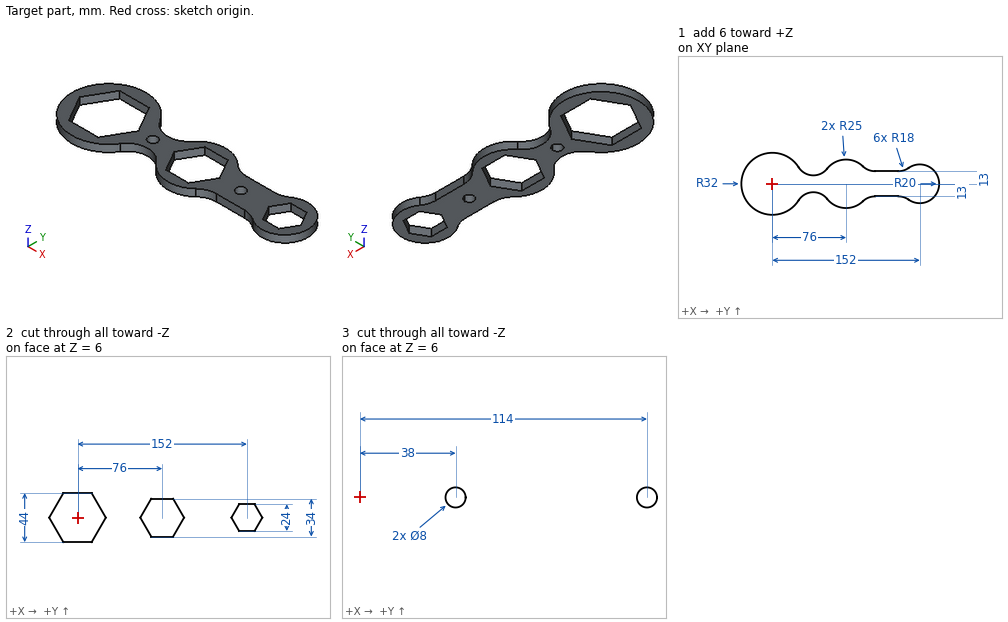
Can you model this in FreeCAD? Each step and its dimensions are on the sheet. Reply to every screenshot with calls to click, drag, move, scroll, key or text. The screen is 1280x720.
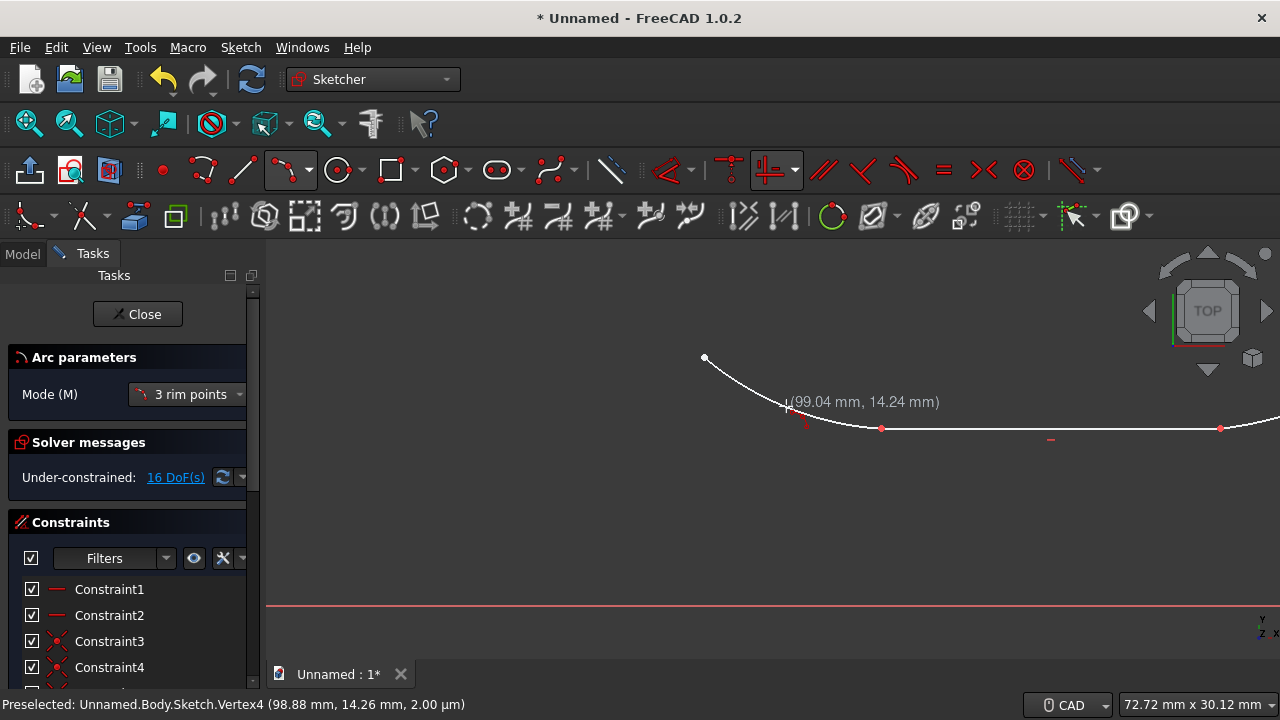
scroll(786, 409, down, 8)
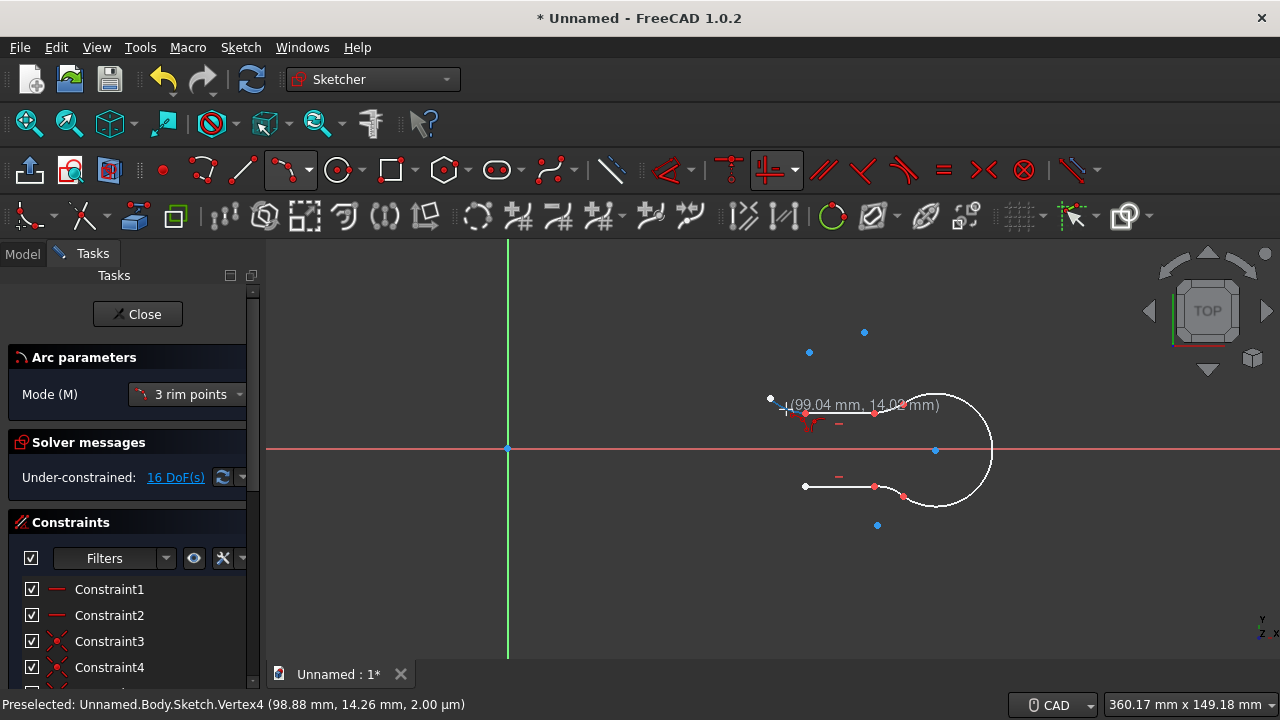
click(770, 399)
click(666, 405)
click(717, 379)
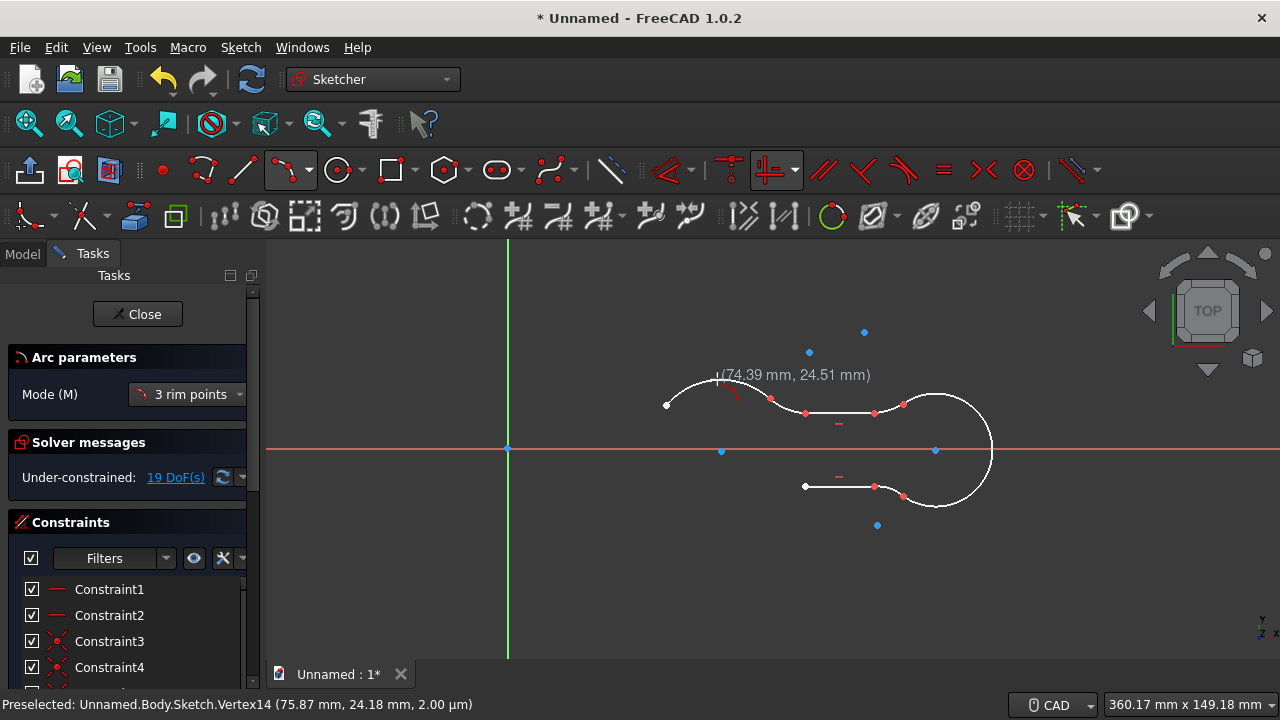
click(666, 406)
click(584, 401)
click(624, 424)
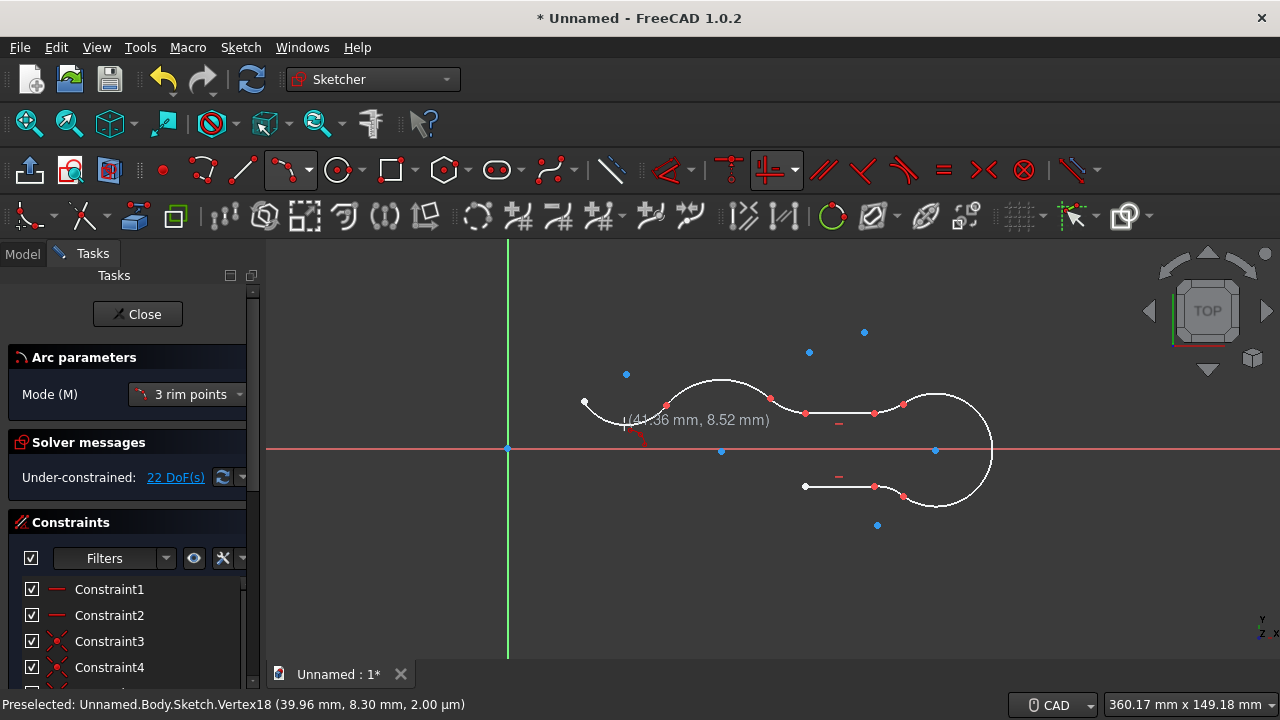
click(584, 402)
click(584, 497)
click(429, 405)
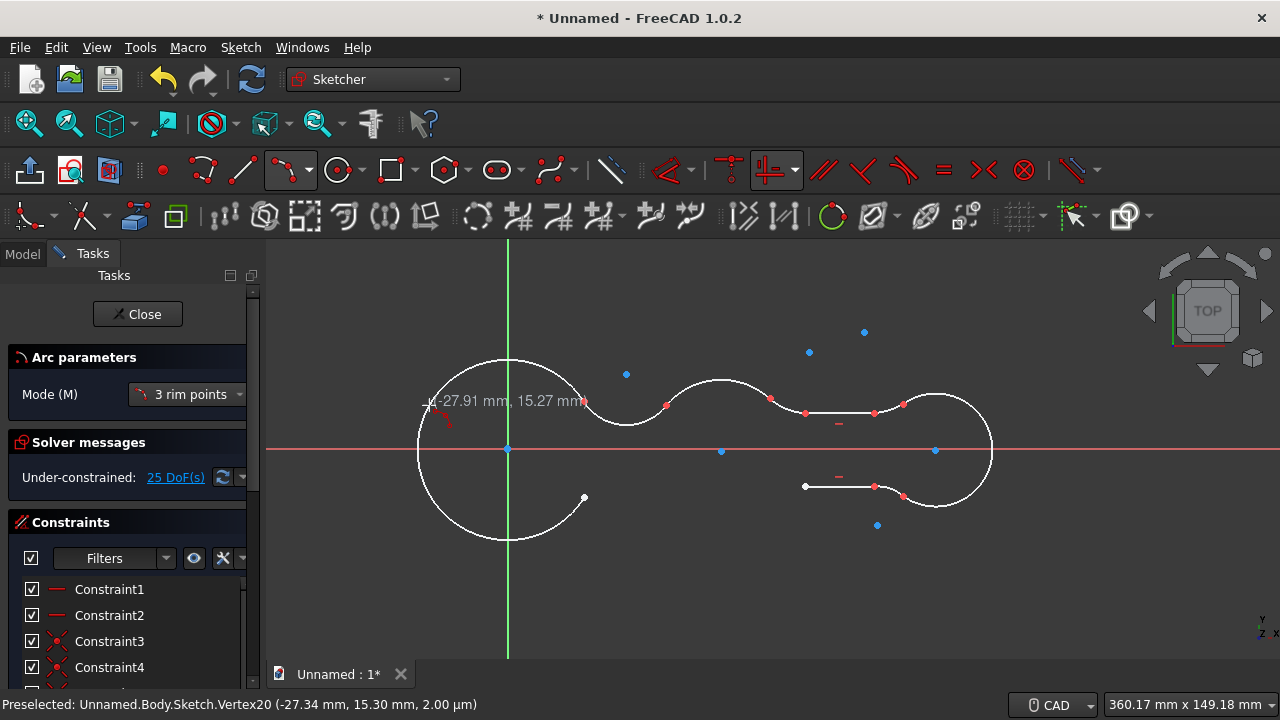
click(584, 498)
click(666, 493)
click(624, 474)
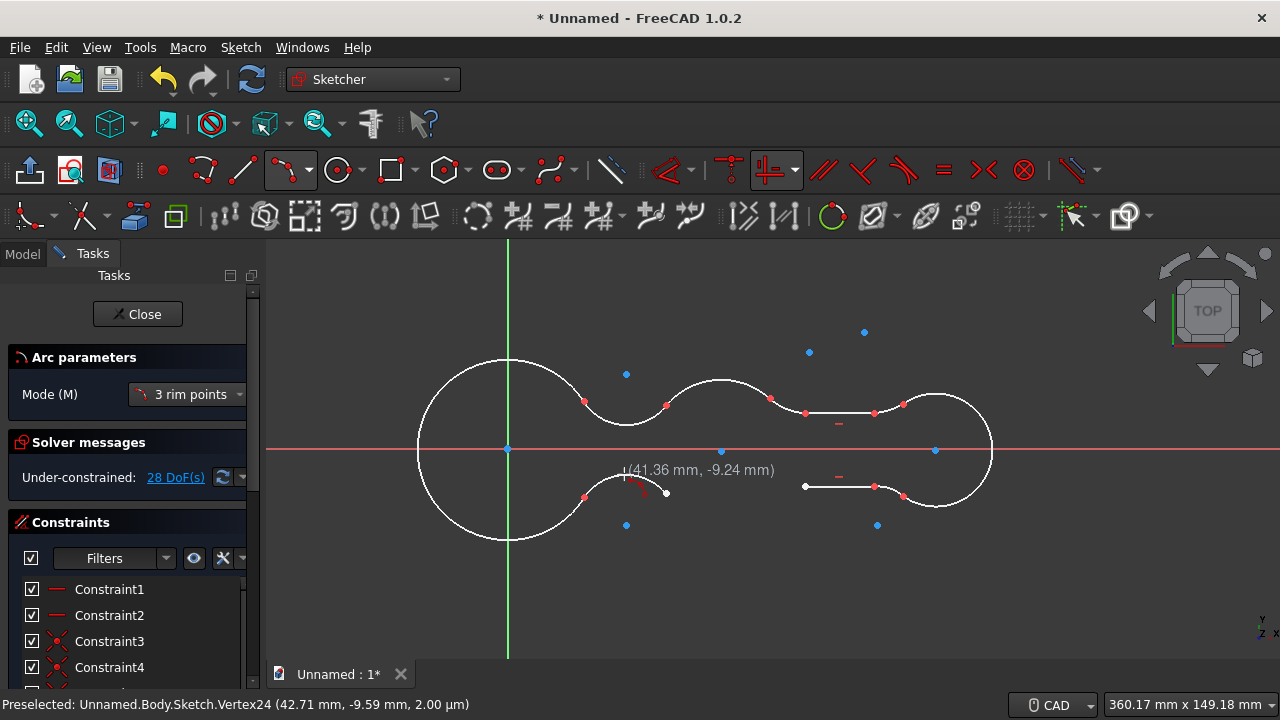
click(666, 494)
click(770, 500)
click(717, 519)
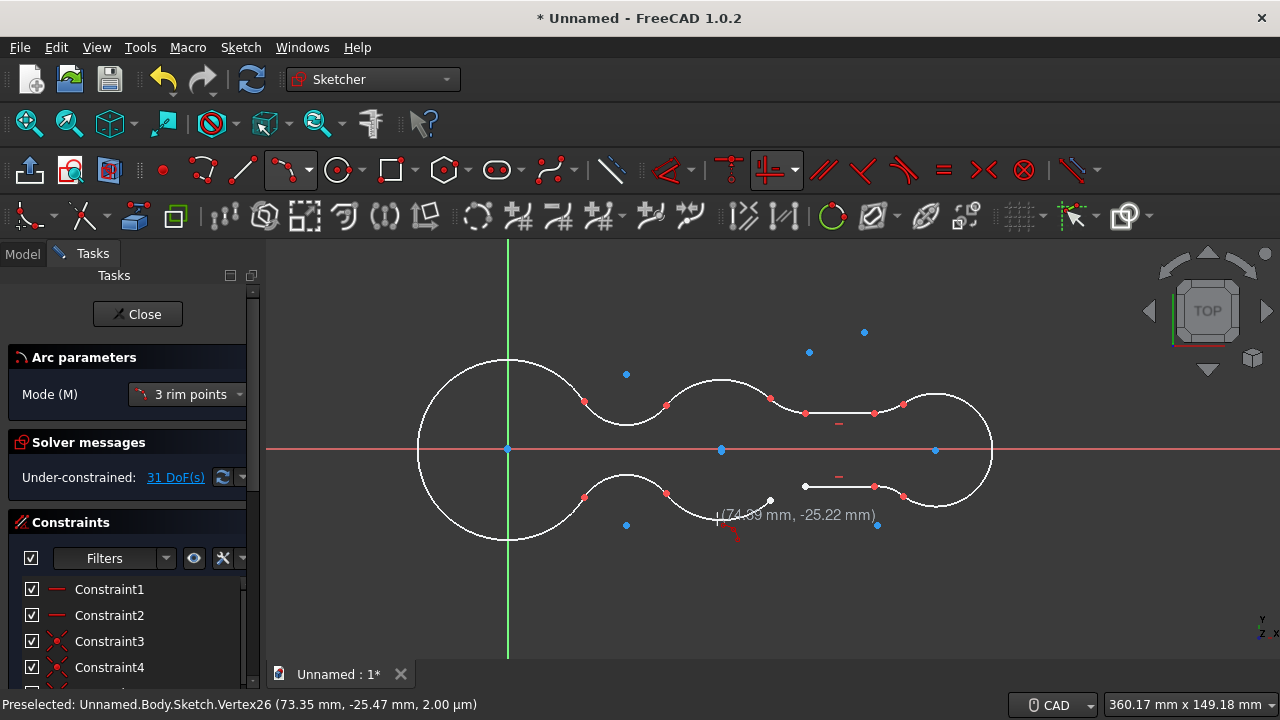
click(770, 501)
click(806, 487)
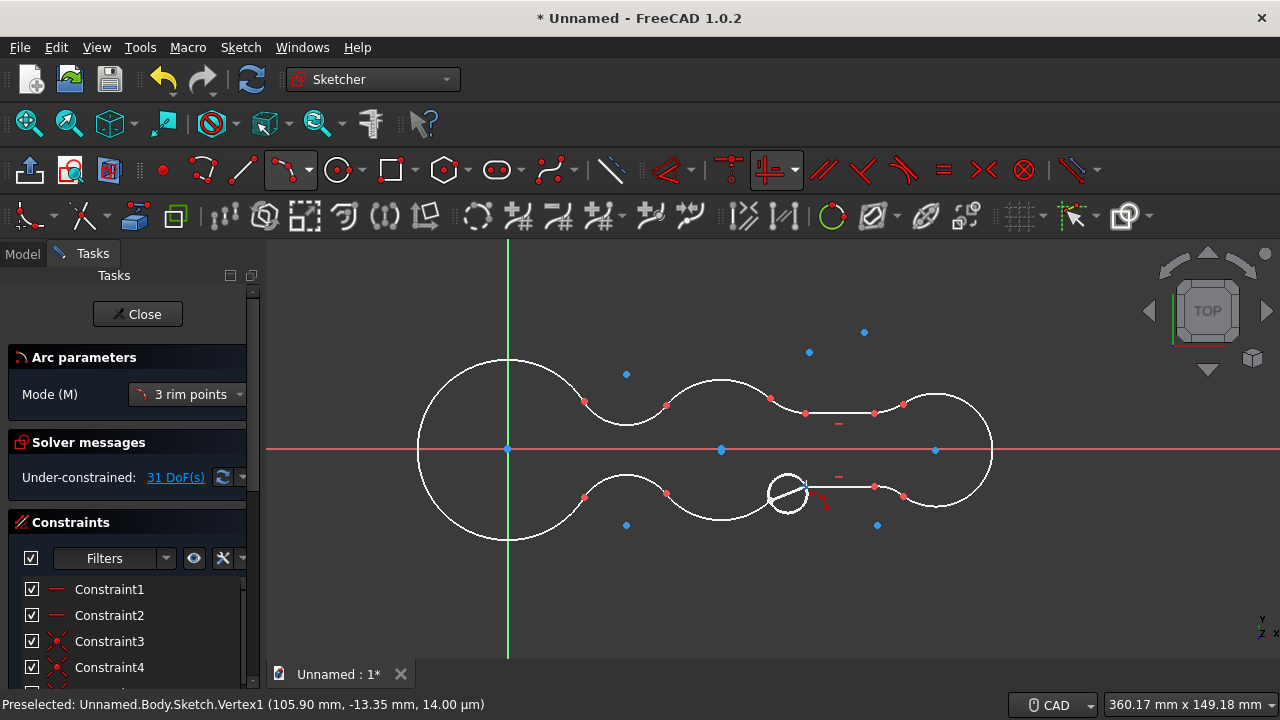
scroll(786, 489, up, 8)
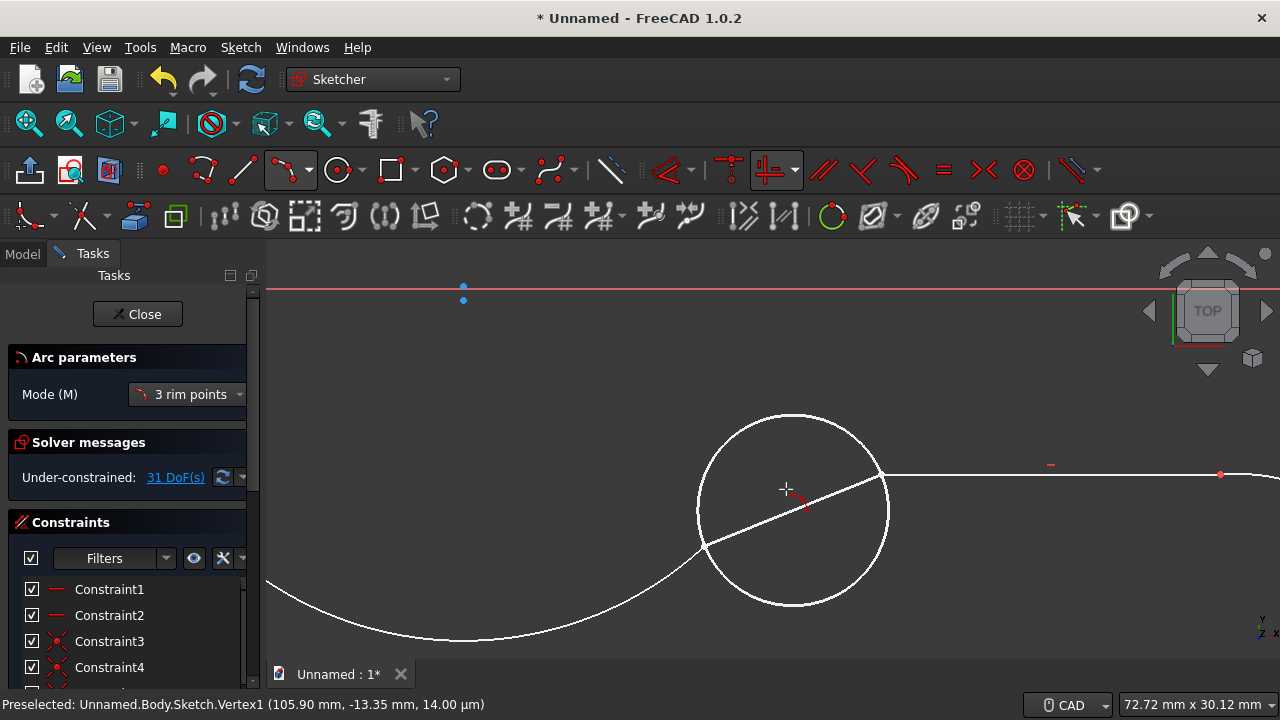
click(786, 488)
key(Escape)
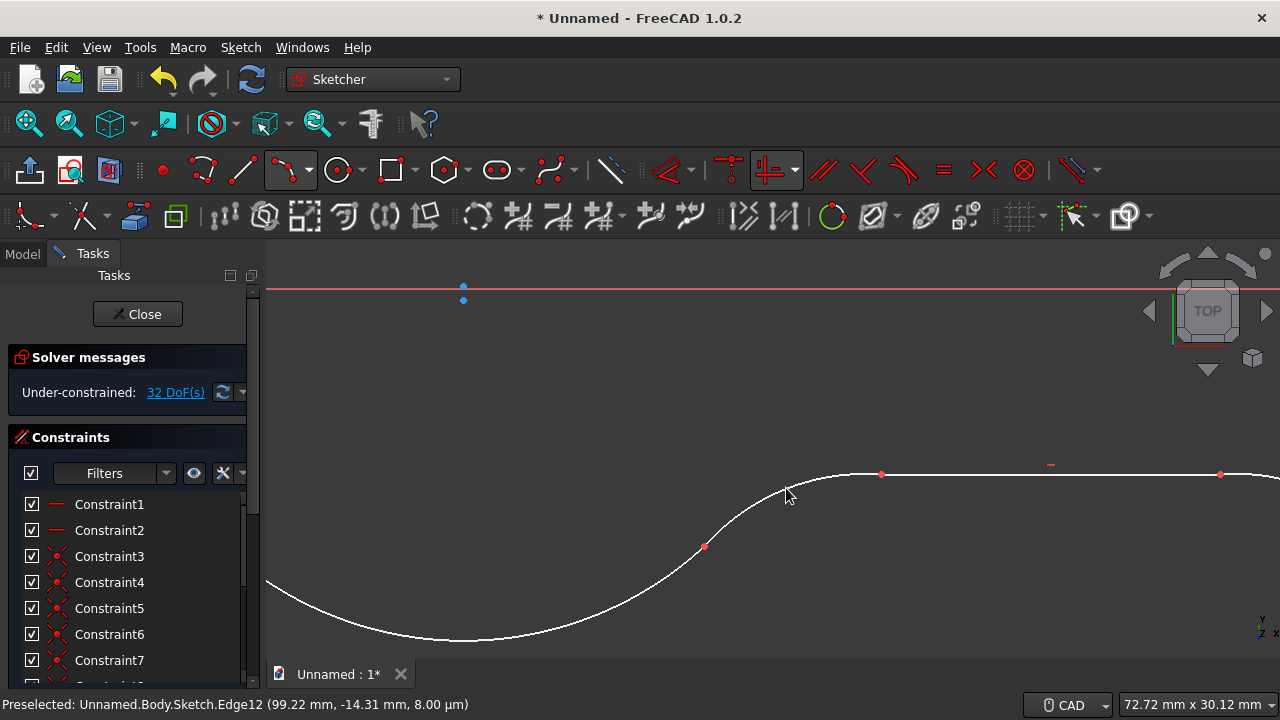
scroll(786, 490, down, 8)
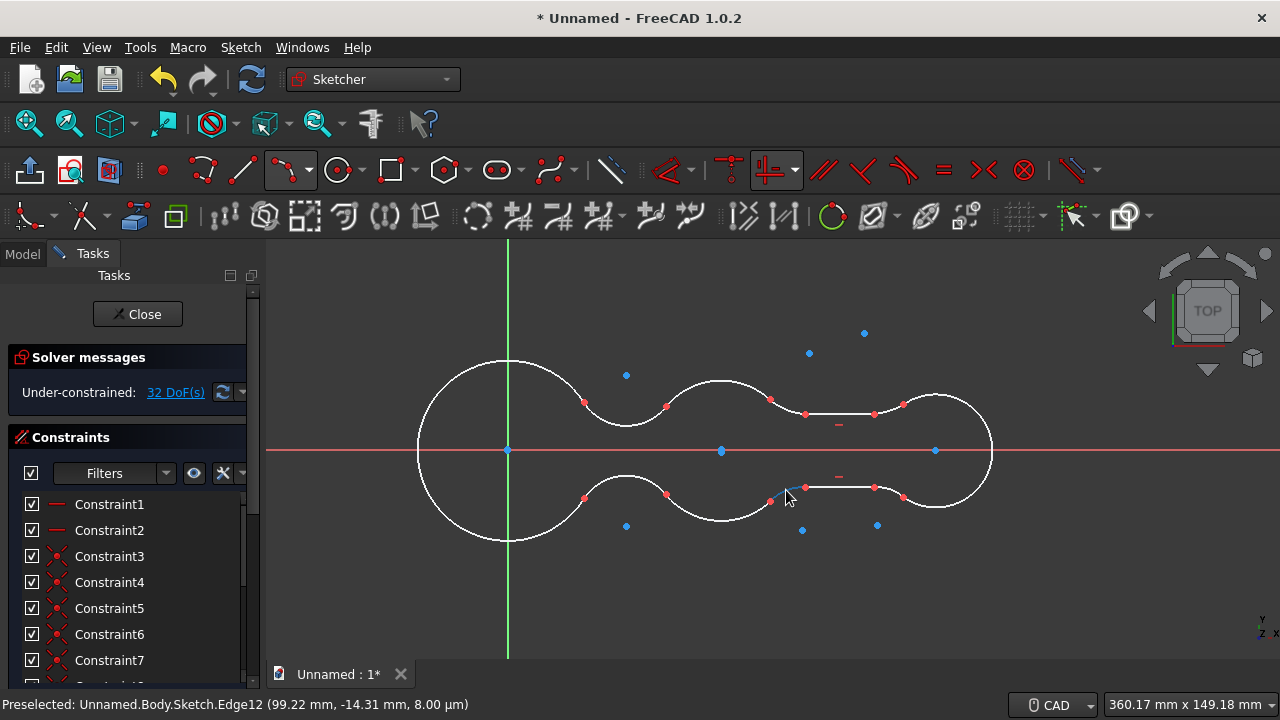
click(826, 487)